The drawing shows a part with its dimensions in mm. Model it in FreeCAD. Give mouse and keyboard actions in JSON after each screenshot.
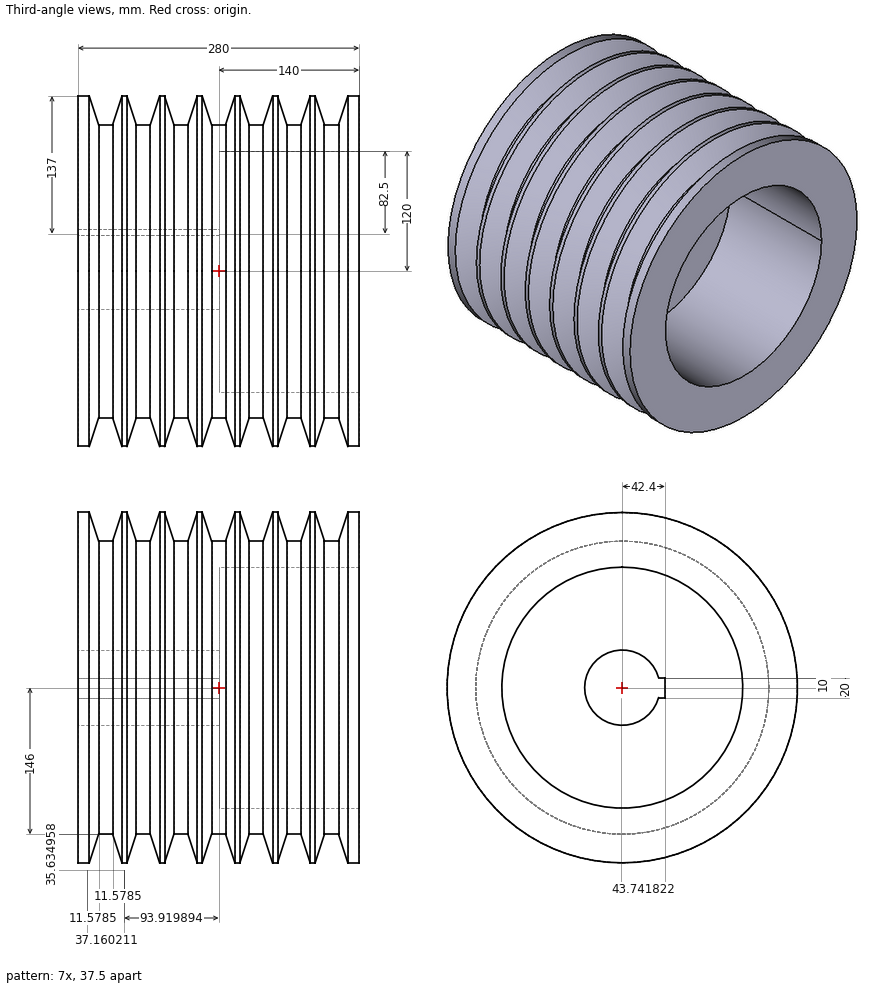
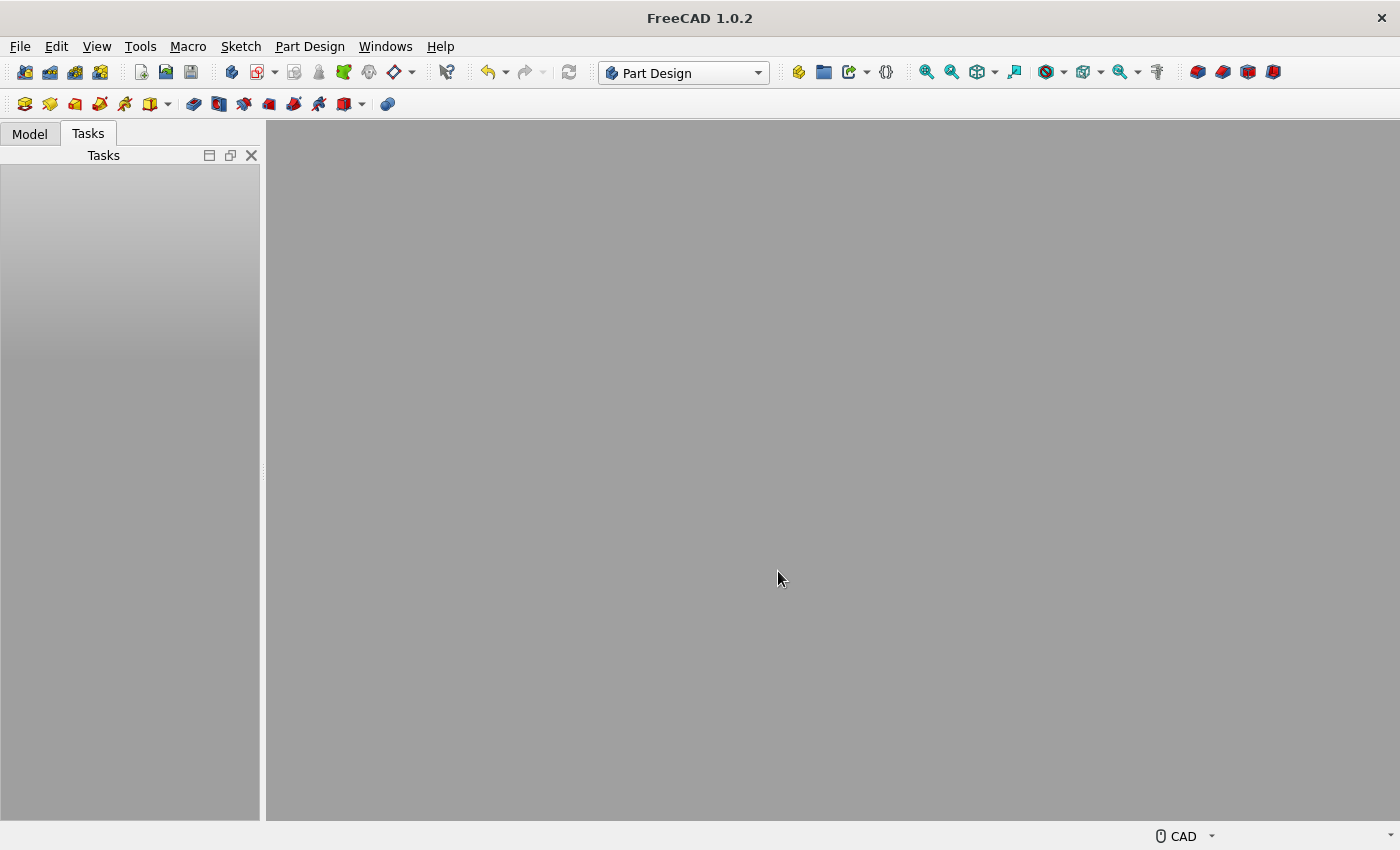
{"action": "left_click", "coordinate": [141, 72]}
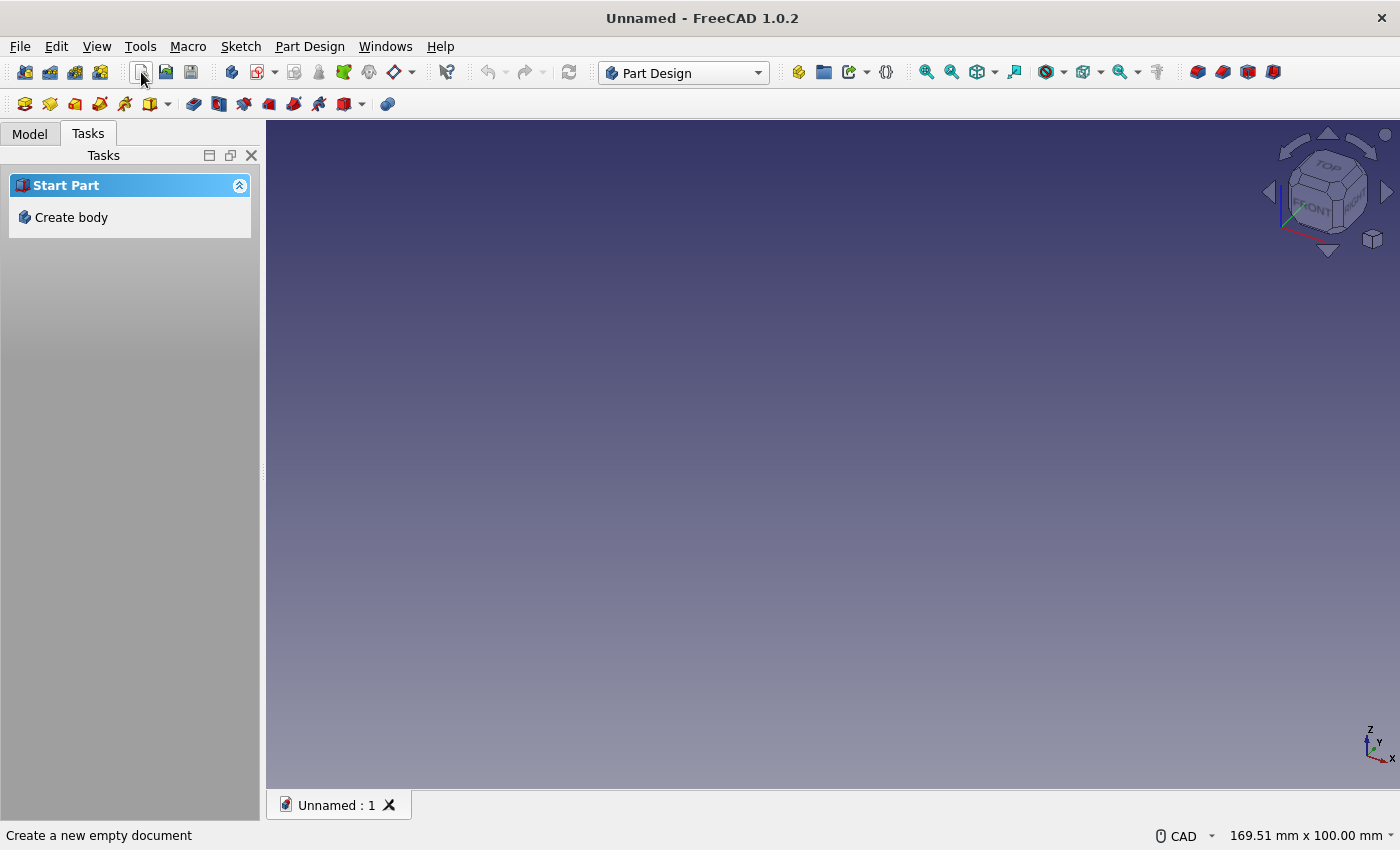
{"action": "left_click", "coordinate": [256, 72]}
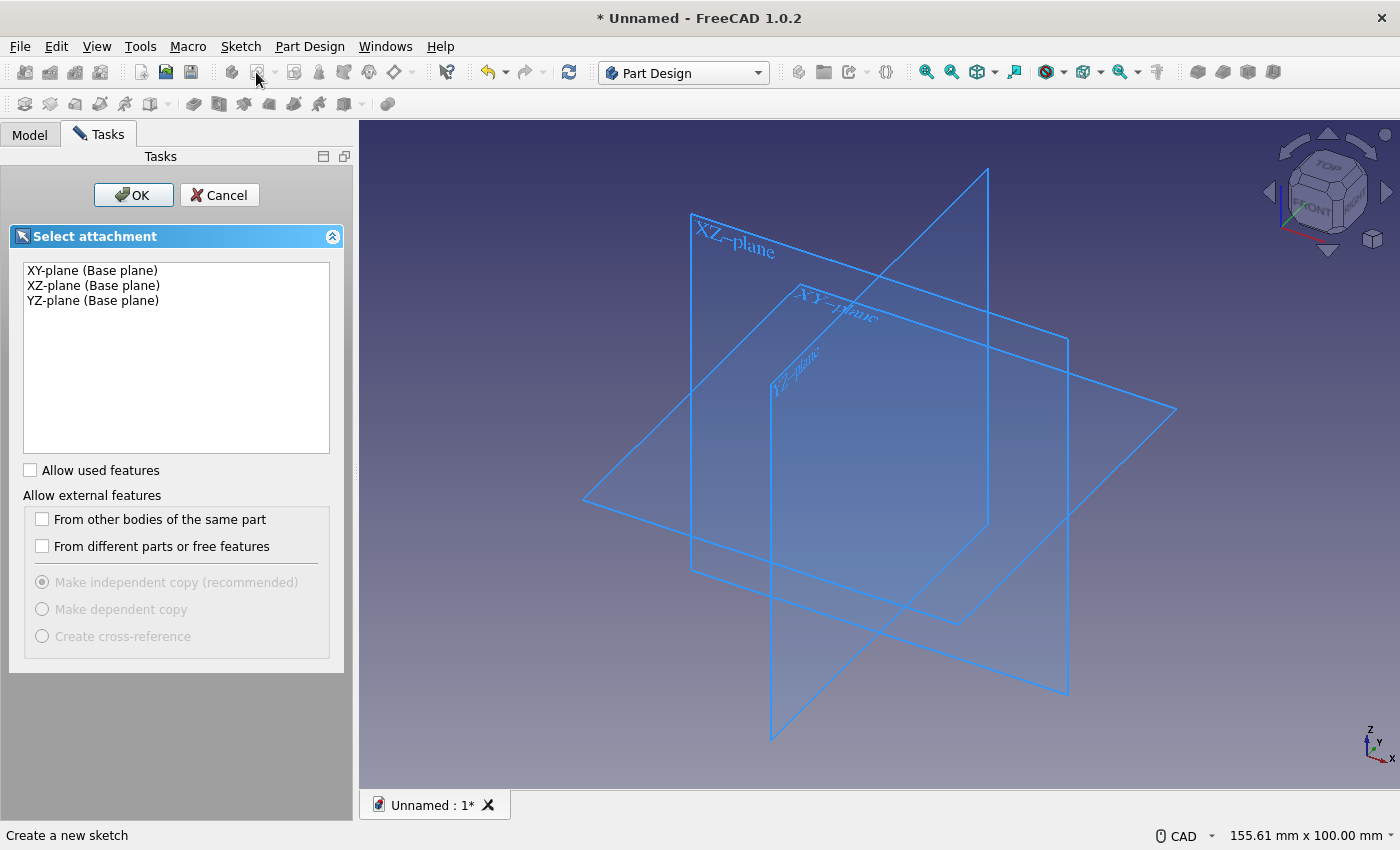
{"action": "left_click", "coordinate": [84, 270]}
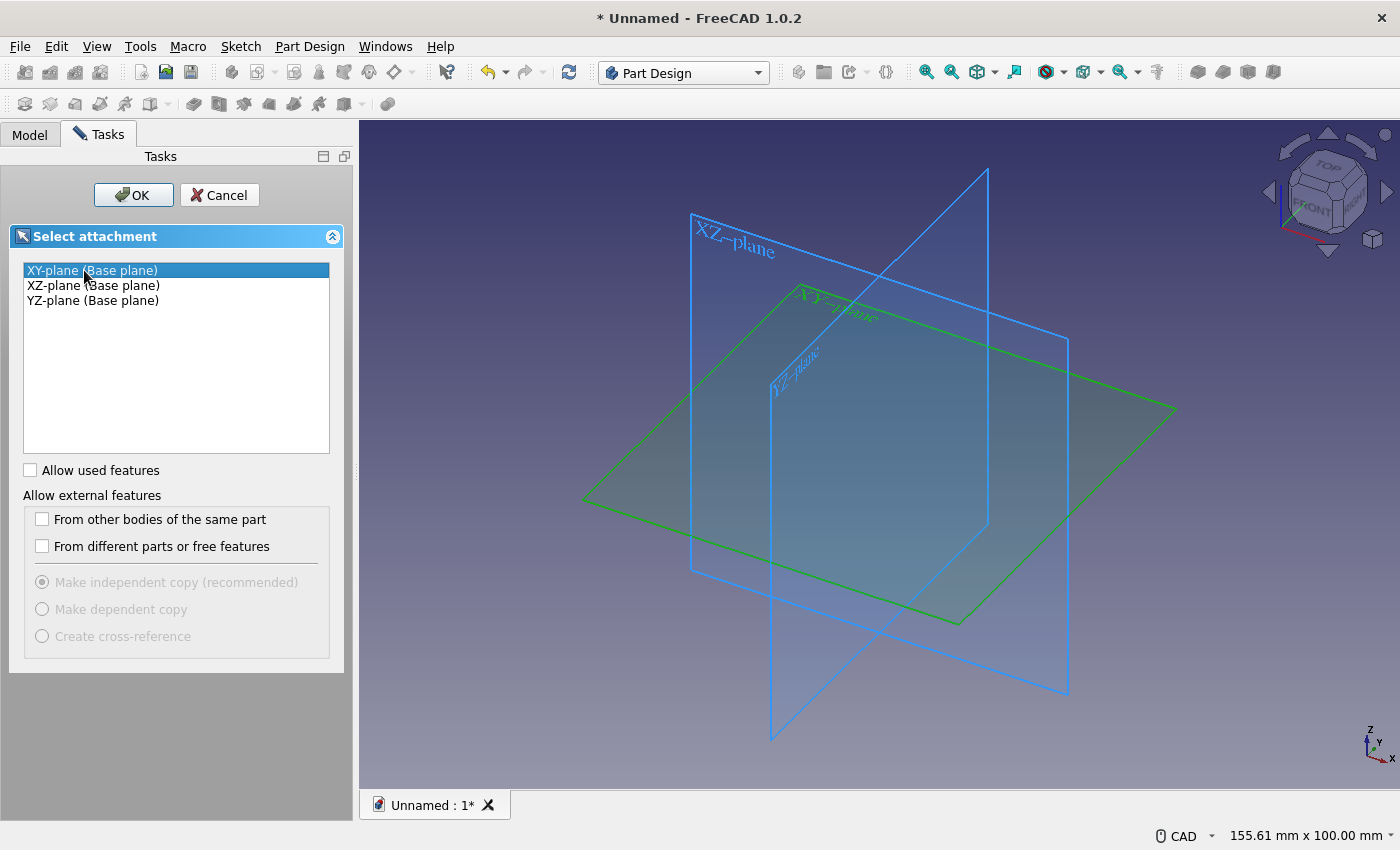
{"action": "left_click", "coordinate": [134, 195]}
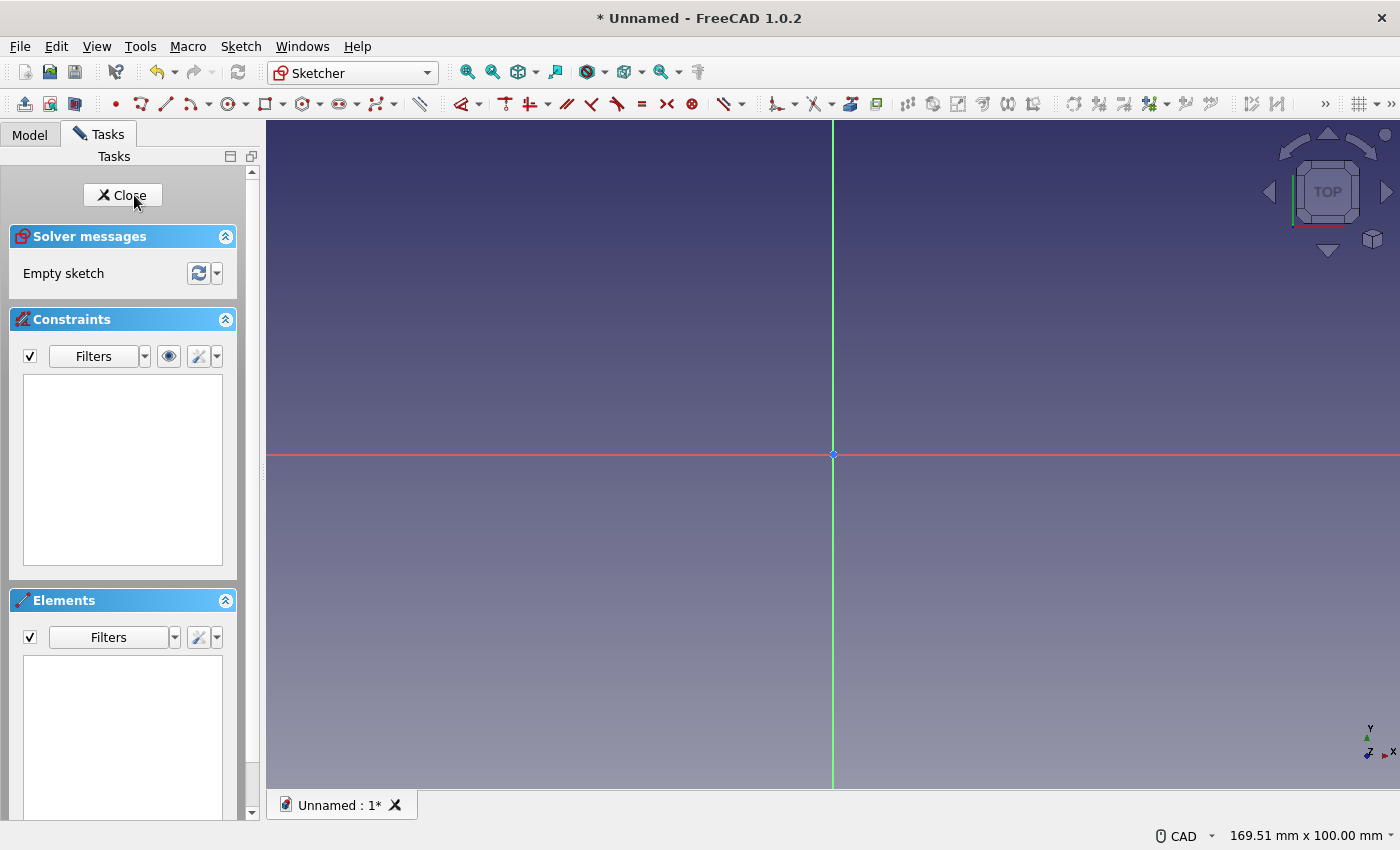
{"action": "scroll", "coordinate": [725, 761], "scroll_direction": "down", "scroll_amount": 5}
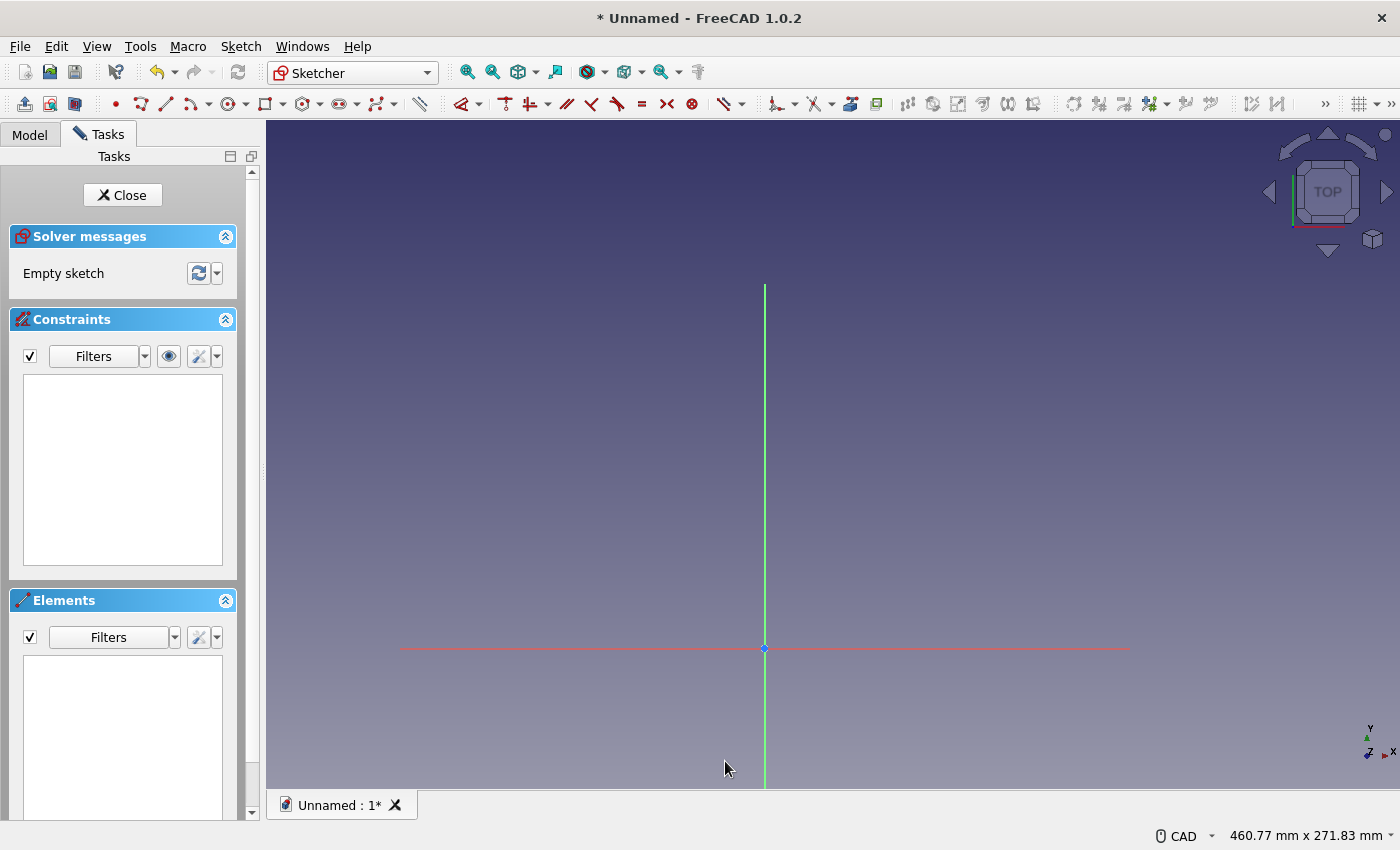
{"action": "left_click", "coordinate": [141, 104]}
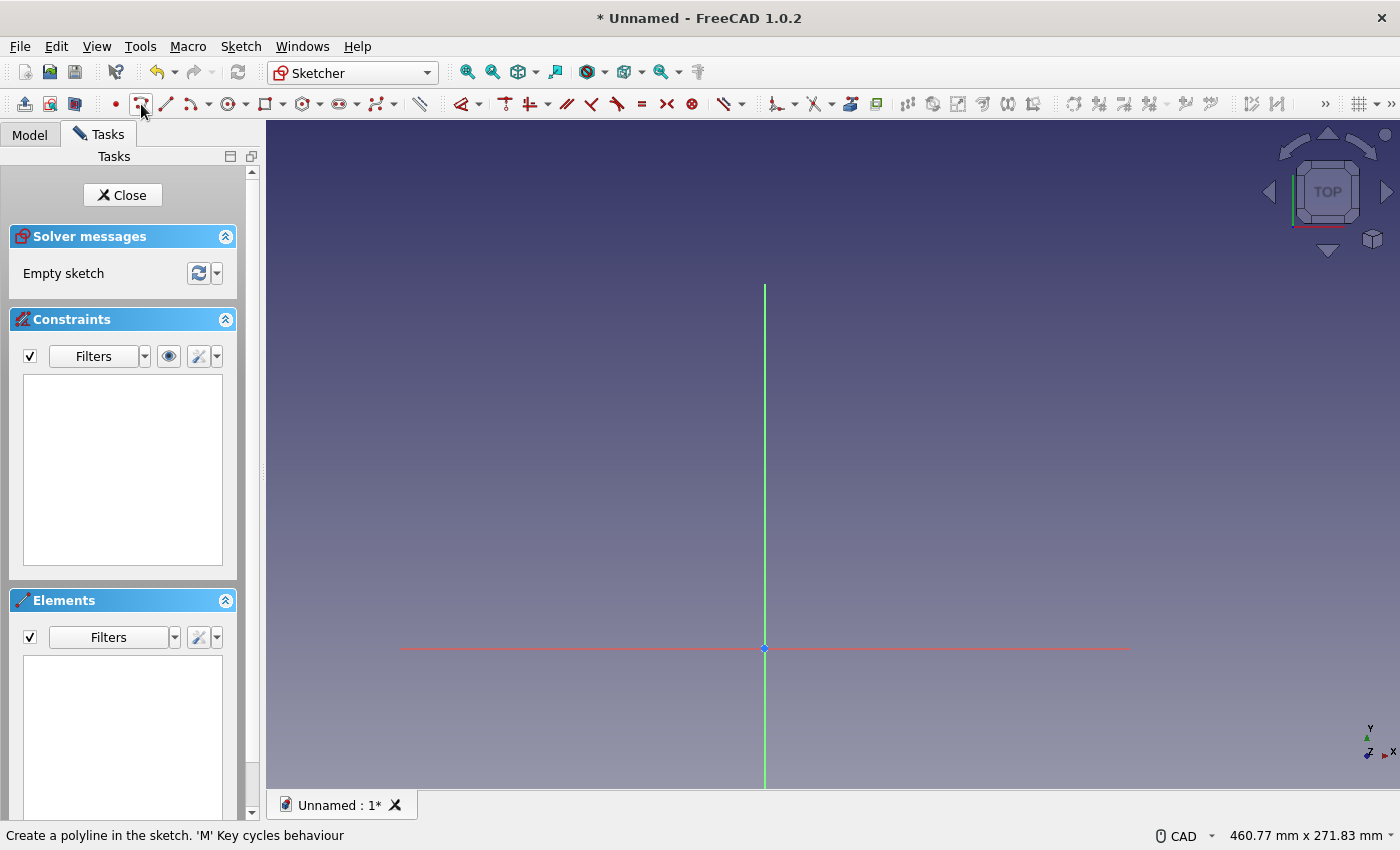
{"action": "left_click", "coordinate": [765, 557]}
{"action": "left_click", "coordinate": [774, 354]}
{"action": "left_click", "coordinate": [1110, 354]}
{"action": "left_click", "coordinate": [1110, 219]}
{"action": "left_click", "coordinate": [420, 219]}
{"action": "left_click", "coordinate": [420, 557]}
{"action": "left_click", "coordinate": [765, 558]}
{"action": "key", "text": "Escape"}
{"action": "key", "text": "Escape"}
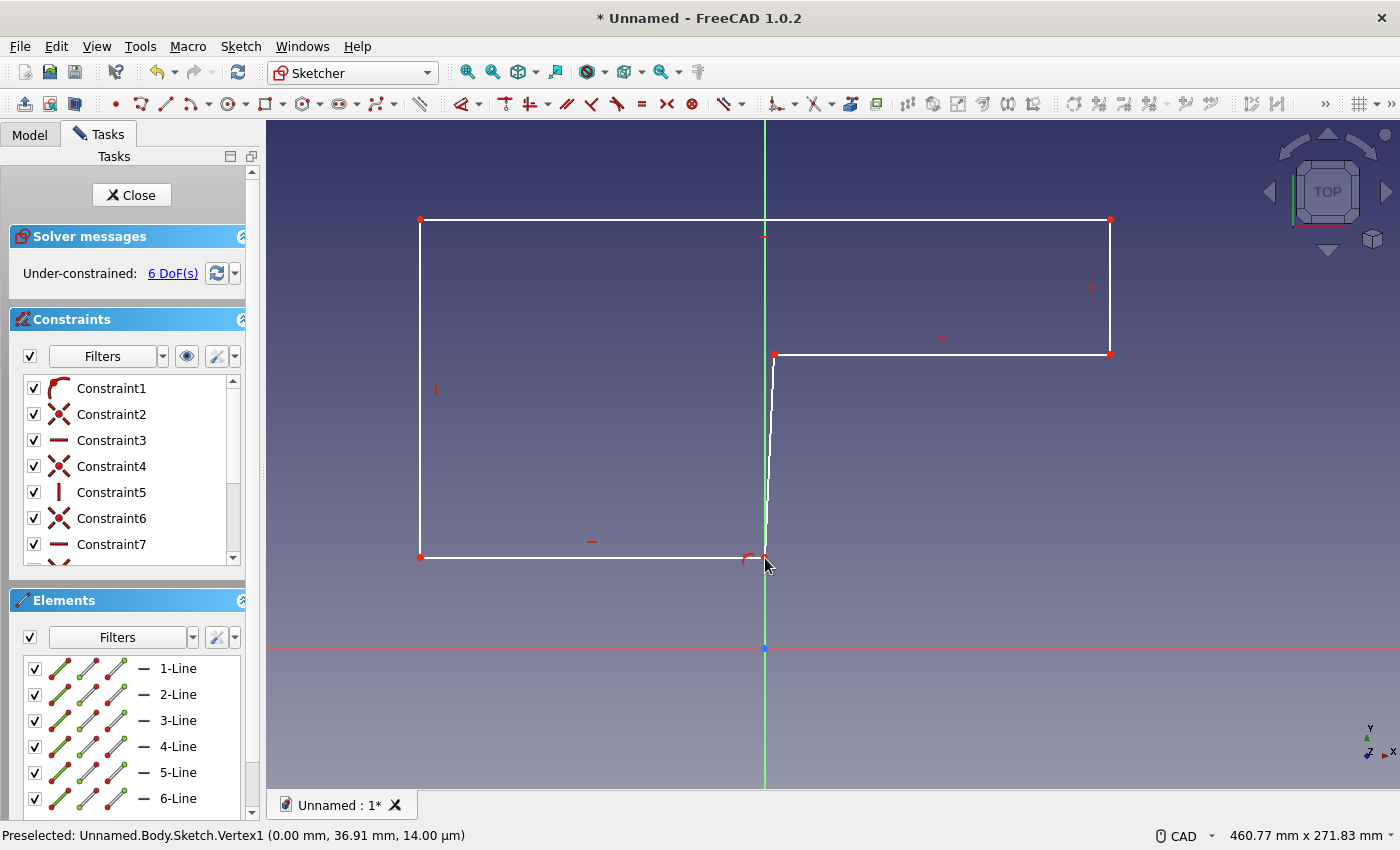
{"action": "left_click", "coordinate": [768, 497]}